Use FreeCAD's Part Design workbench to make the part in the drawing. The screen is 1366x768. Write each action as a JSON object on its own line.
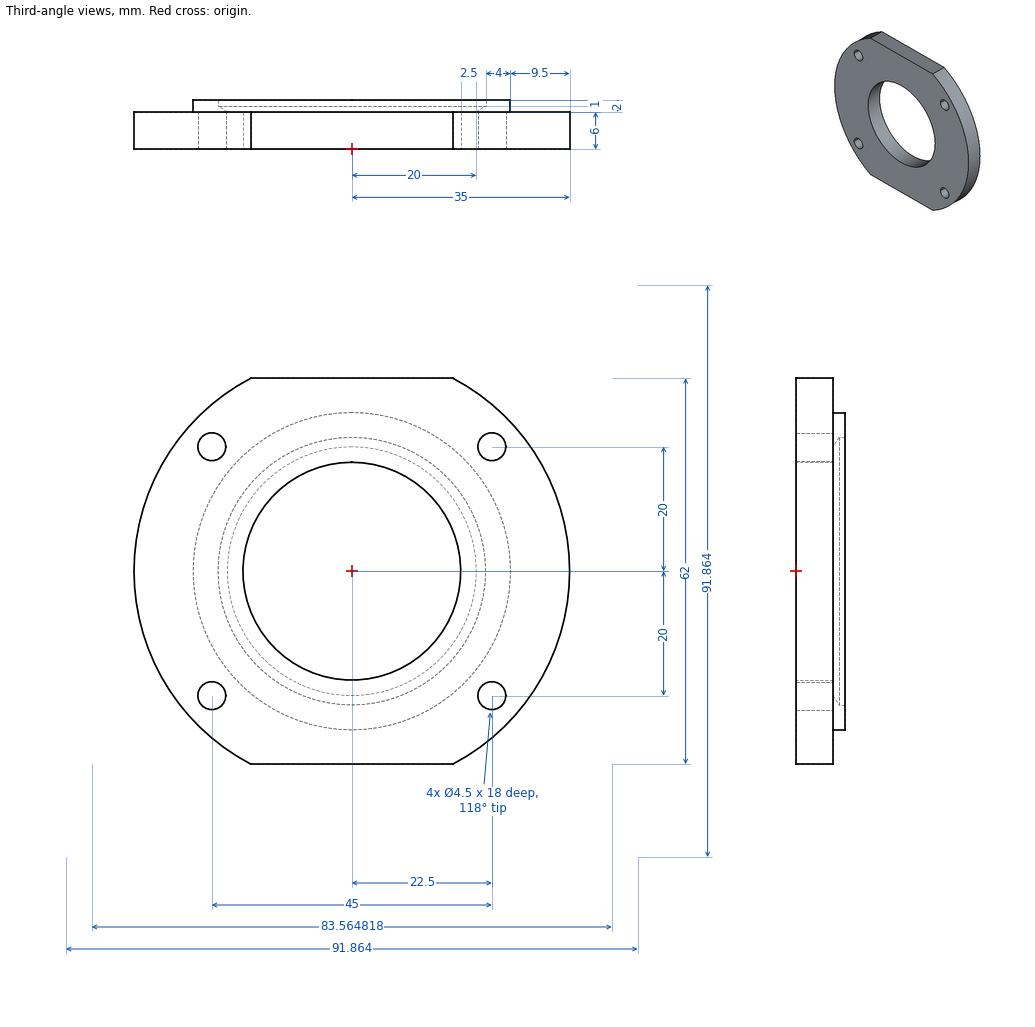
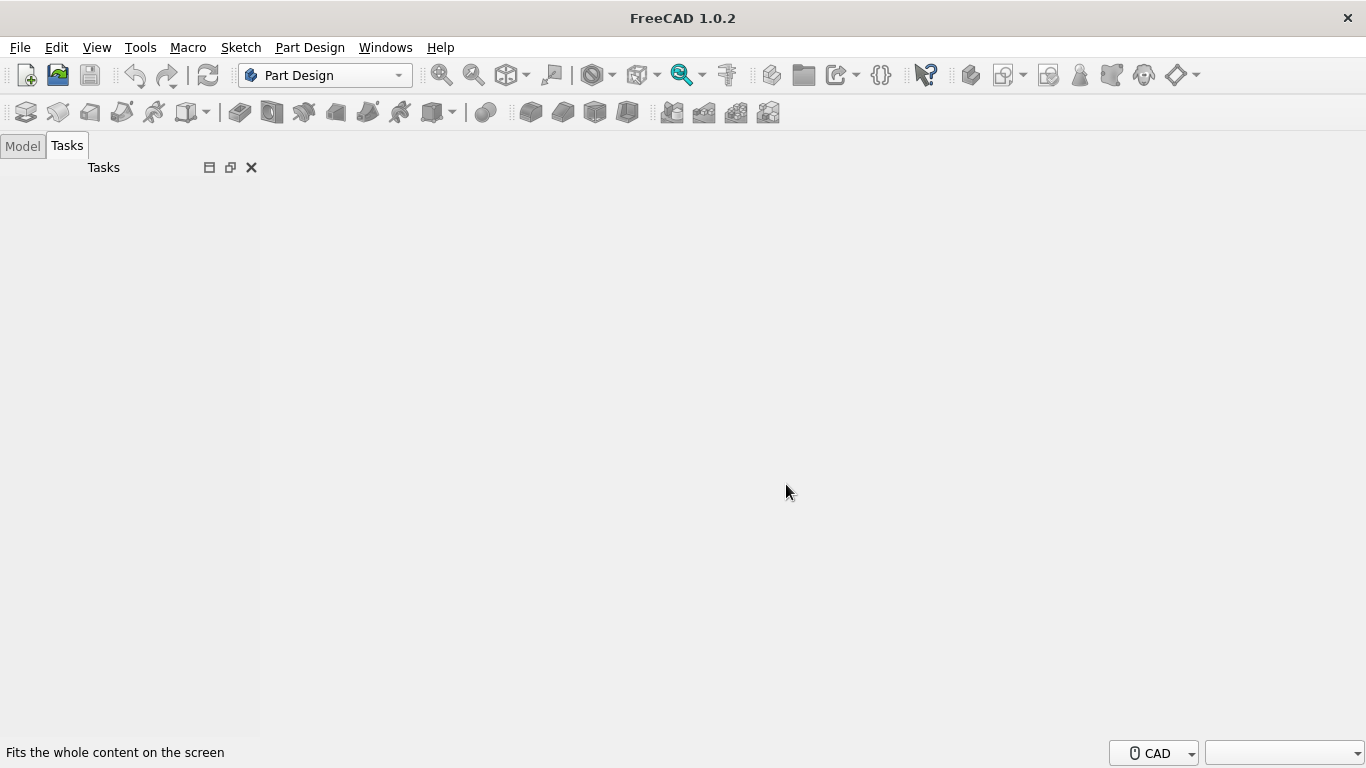
{"action": "left_click", "coordinate": [26, 76]}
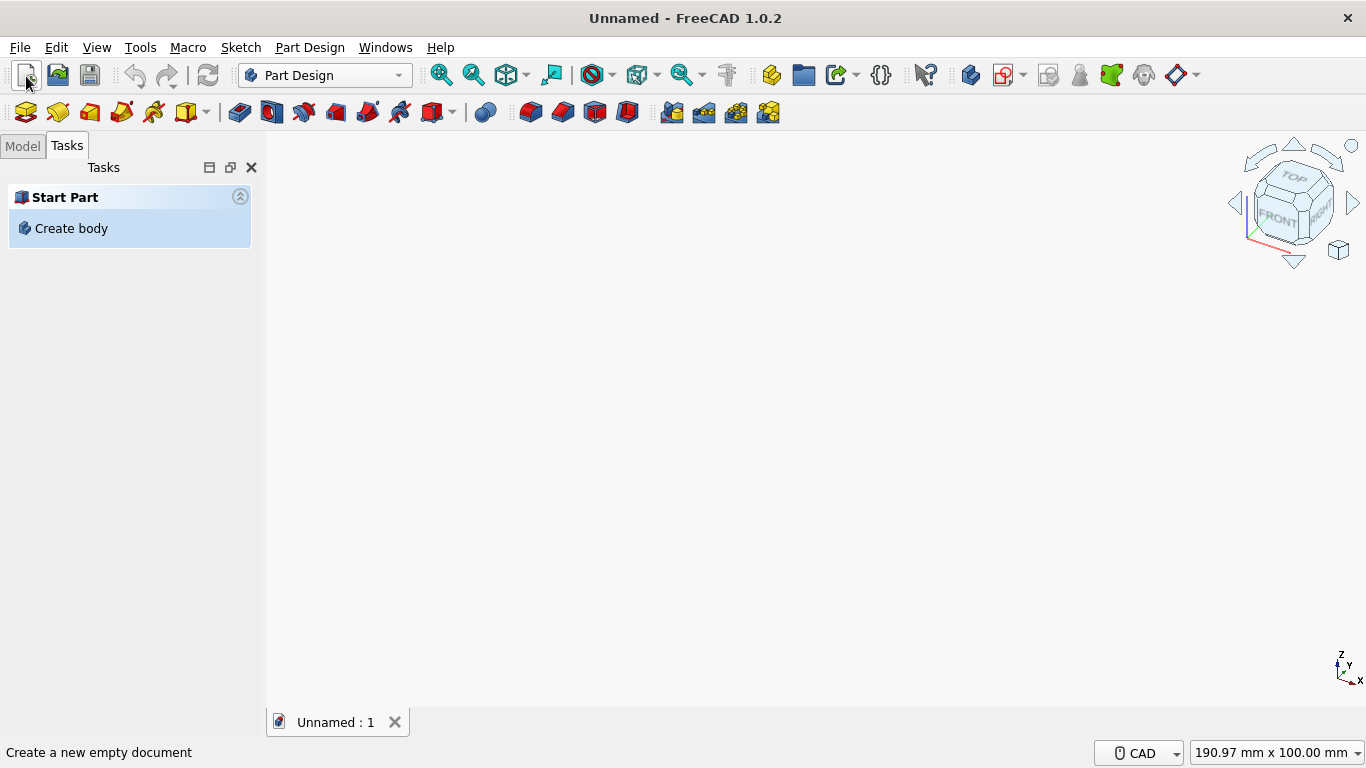
{"action": "left_click", "coordinate": [1004, 76]}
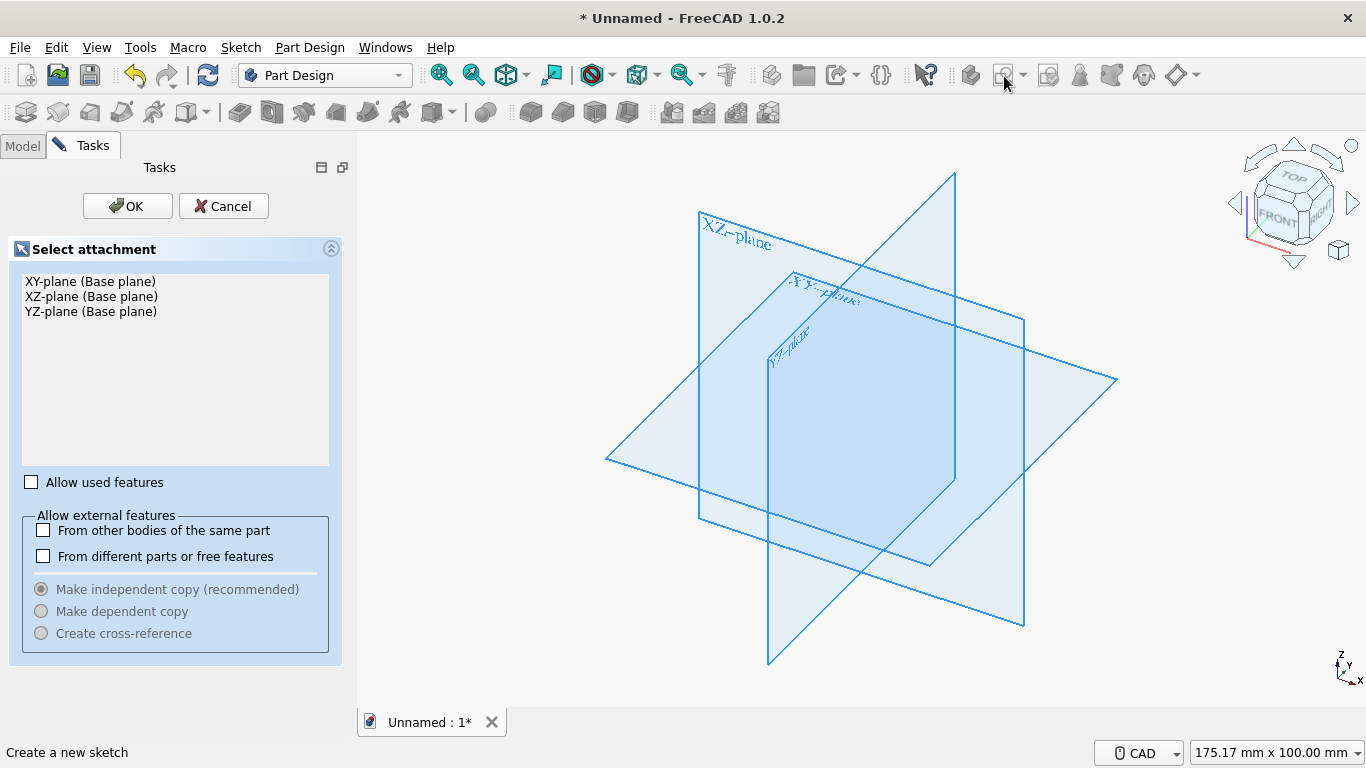
{"action": "left_click", "coordinate": [82, 282]}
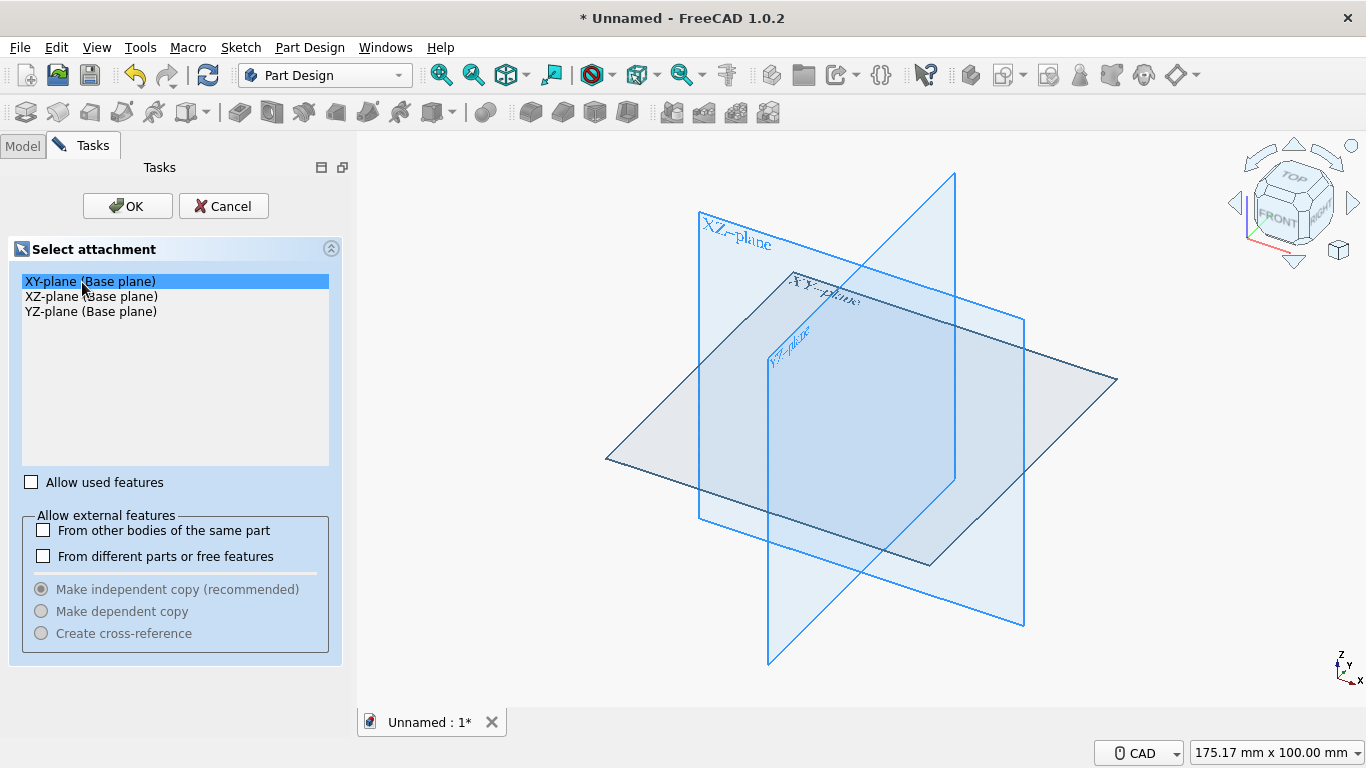
{"action": "left_click", "coordinate": [128, 206]}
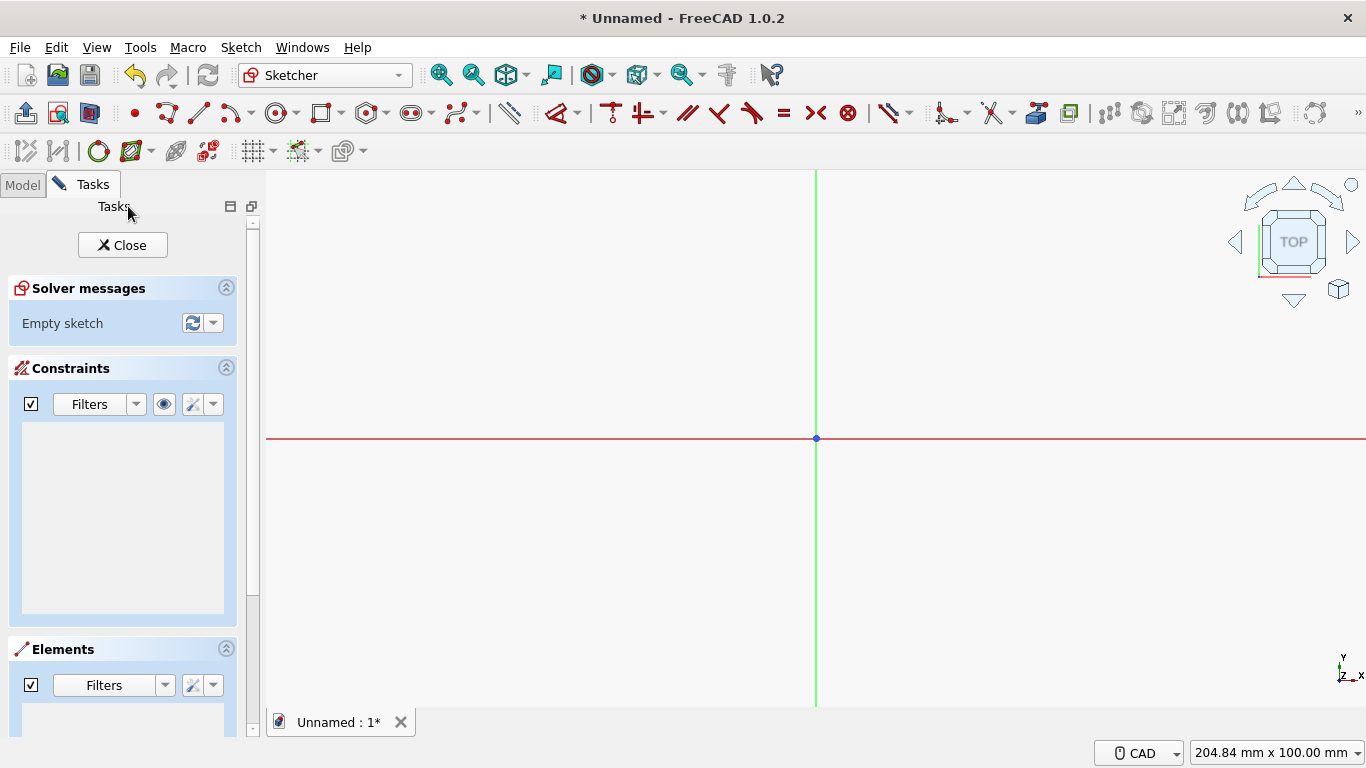
{"action": "scroll", "coordinate": [980, 408], "scroll_direction": "up", "scroll_amount": 6}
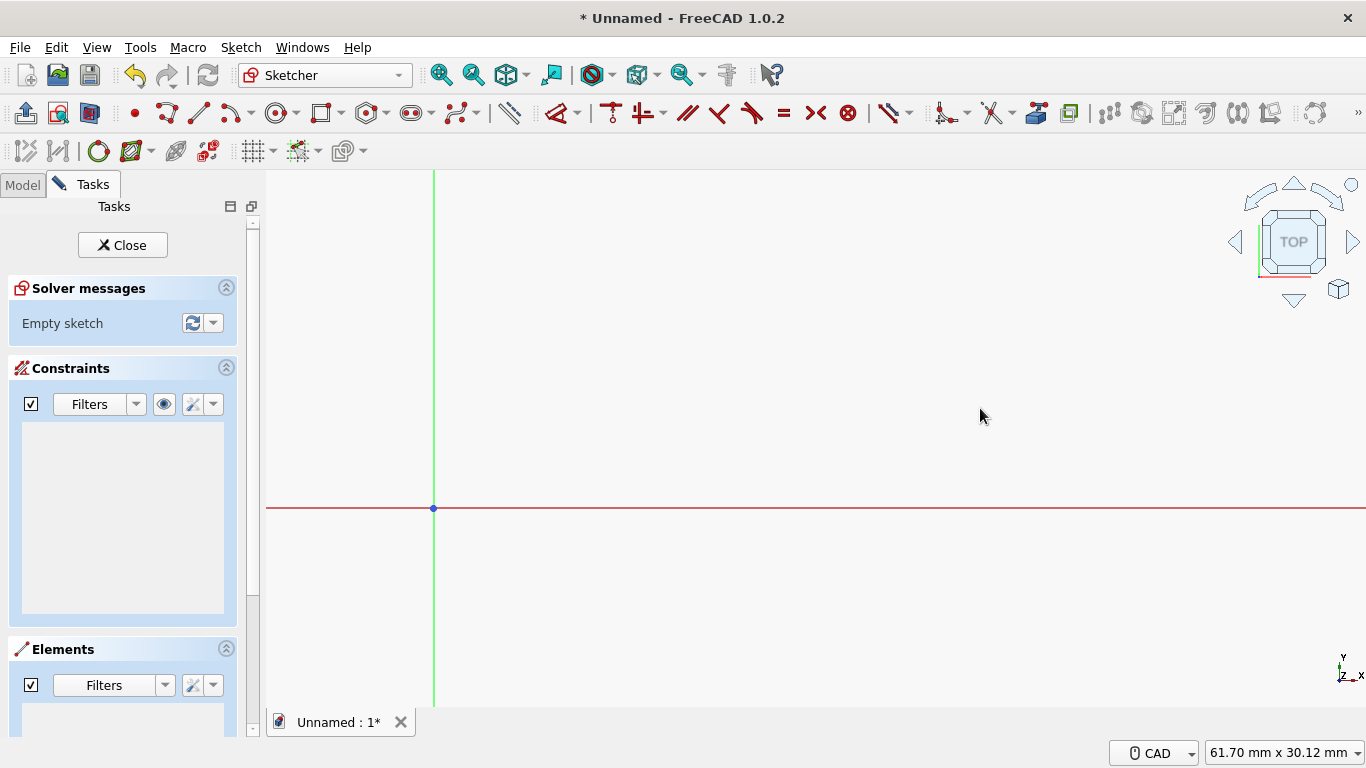
{"action": "left_click", "coordinate": [168, 114]}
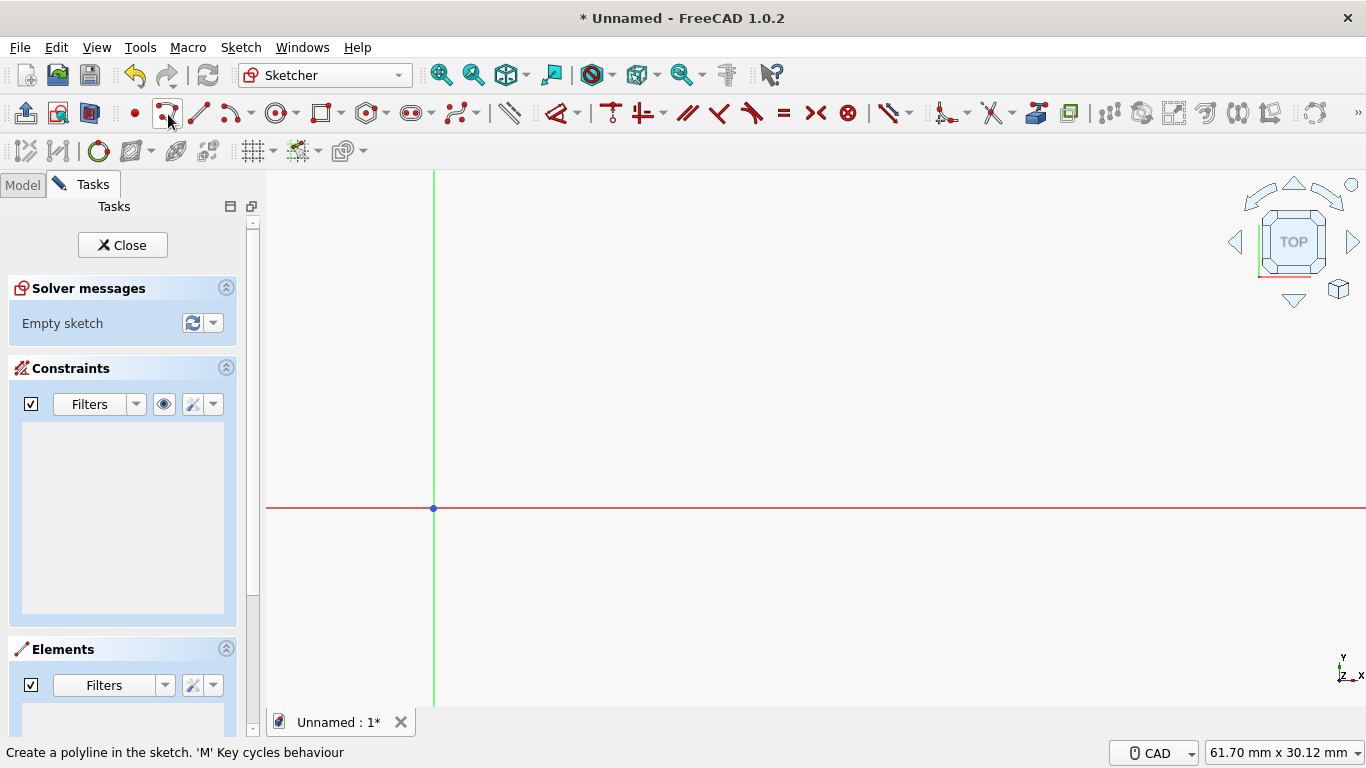
{"action": "left_click", "coordinate": [746, 508]}
{"action": "left_click", "coordinate": [1058, 499]}
{"action": "left_click", "coordinate": [1058, 401]}
{"action": "left_click", "coordinate": [889, 401]}
{"action": "left_click", "coordinate": [889, 366]}
{"action": "left_click", "coordinate": [817, 366]}
{"action": "left_click", "coordinate": [817, 383]}
{"action": "left_click", "coordinate": [791, 401]}
{"action": "left_click", "coordinate": [746, 401]}
{"action": "left_click", "coordinate": [746, 508]}
{"action": "key", "text": "Escape"}
{"action": "key", "text": "Escape"}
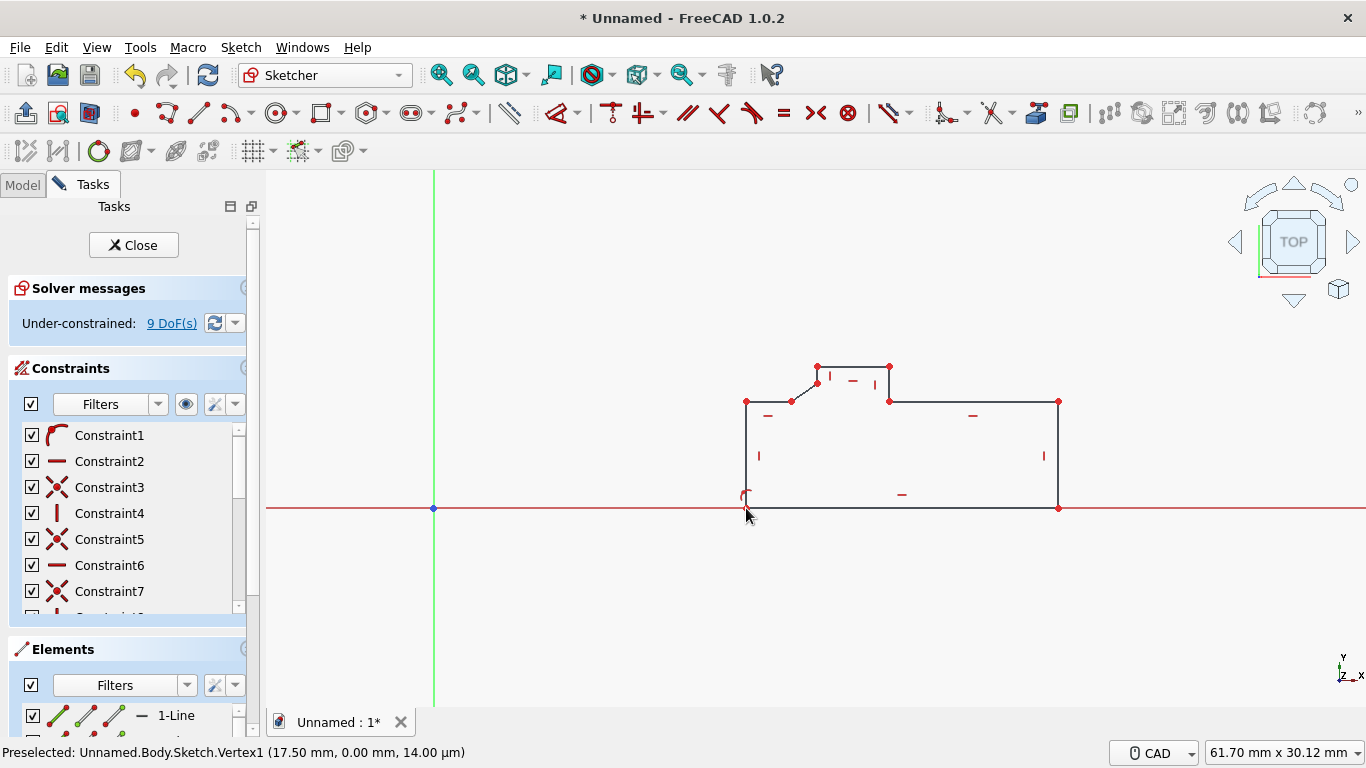
{"action": "left_click", "coordinate": [556, 114]}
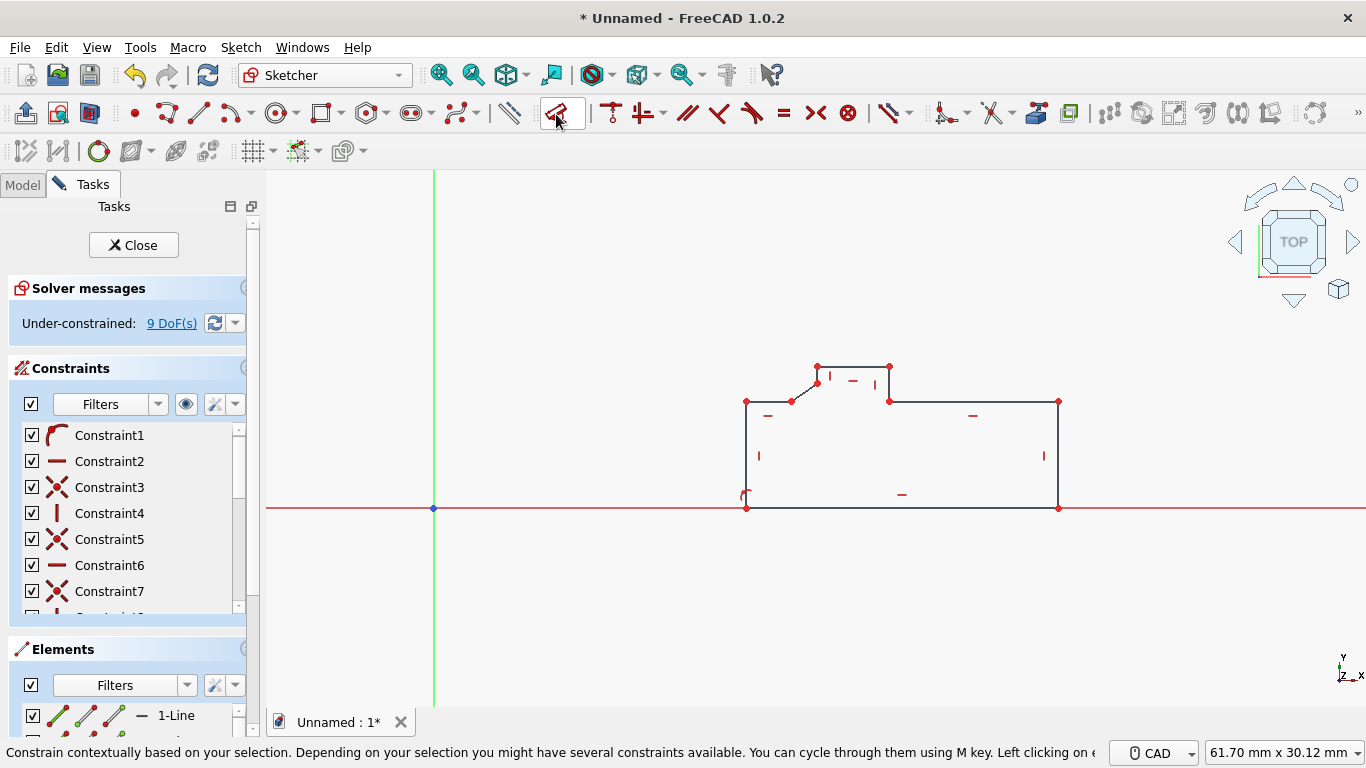
{"action": "left_click", "coordinate": [1058, 476]}
{"action": "left_click", "coordinate": [1092, 455]}